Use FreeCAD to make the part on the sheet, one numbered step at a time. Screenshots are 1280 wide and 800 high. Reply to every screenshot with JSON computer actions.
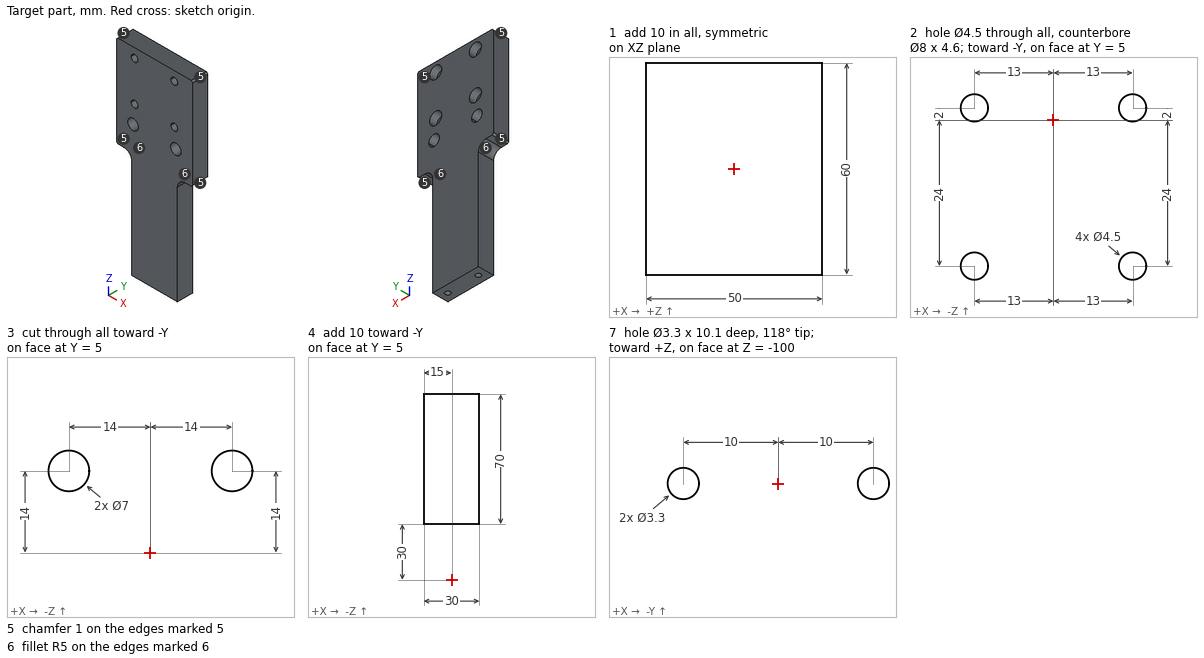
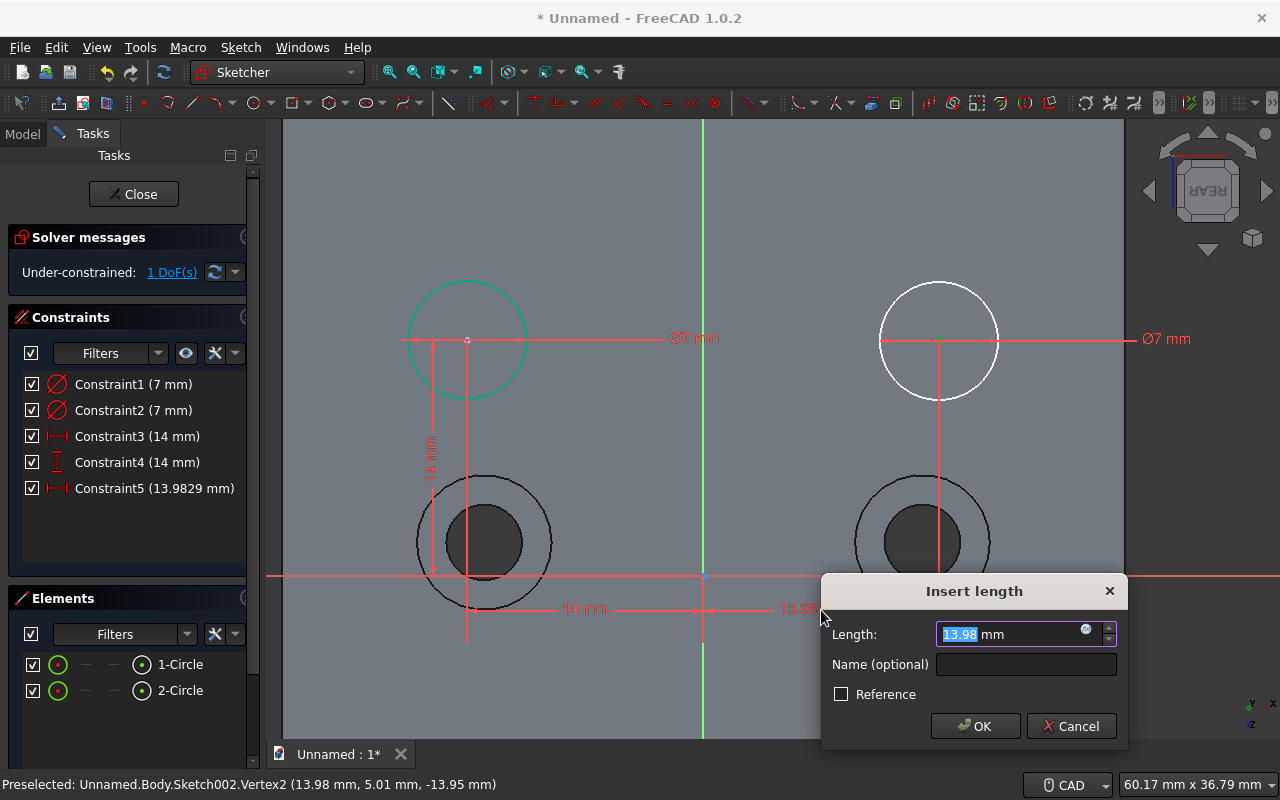
{"action": "type", "text": "14"}
{"action": "key", "text": "Return"}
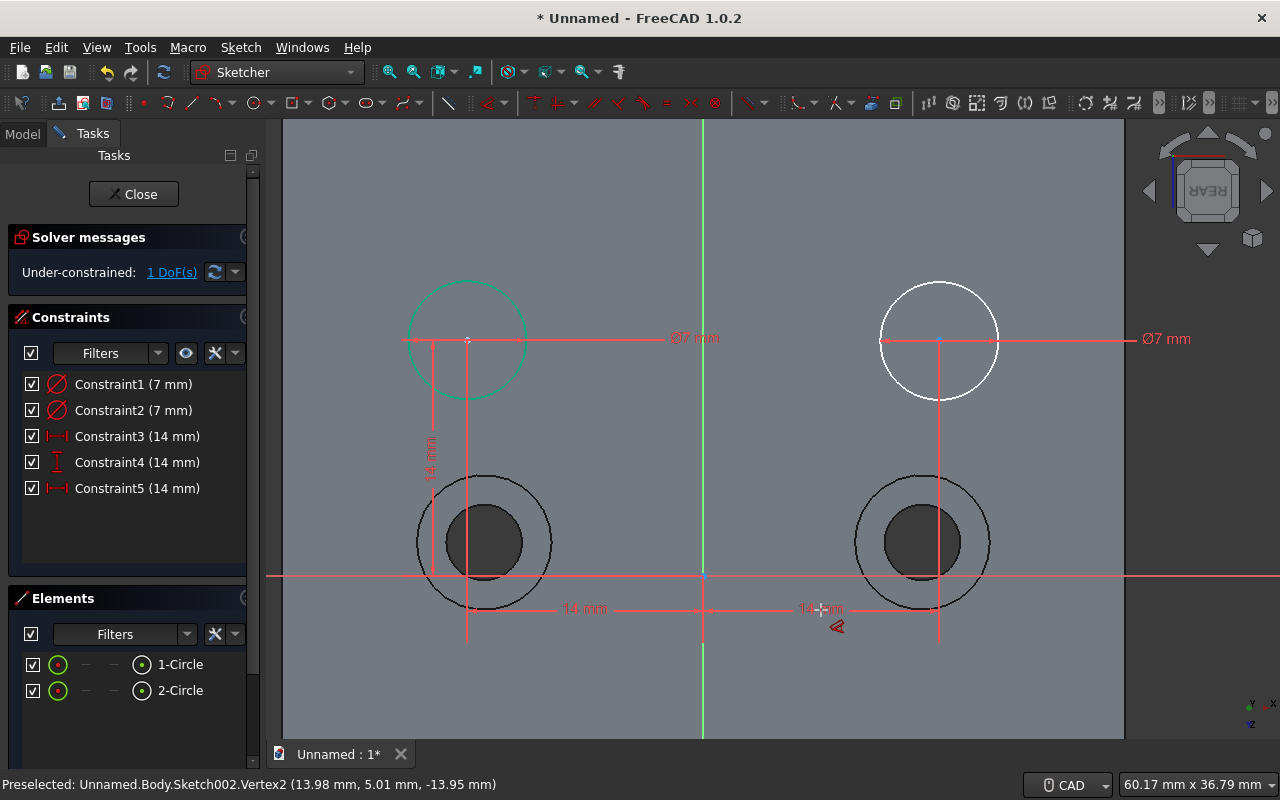
{"action": "left_click", "coordinate": [939, 341]}
{"action": "left_click", "coordinate": [973, 459]}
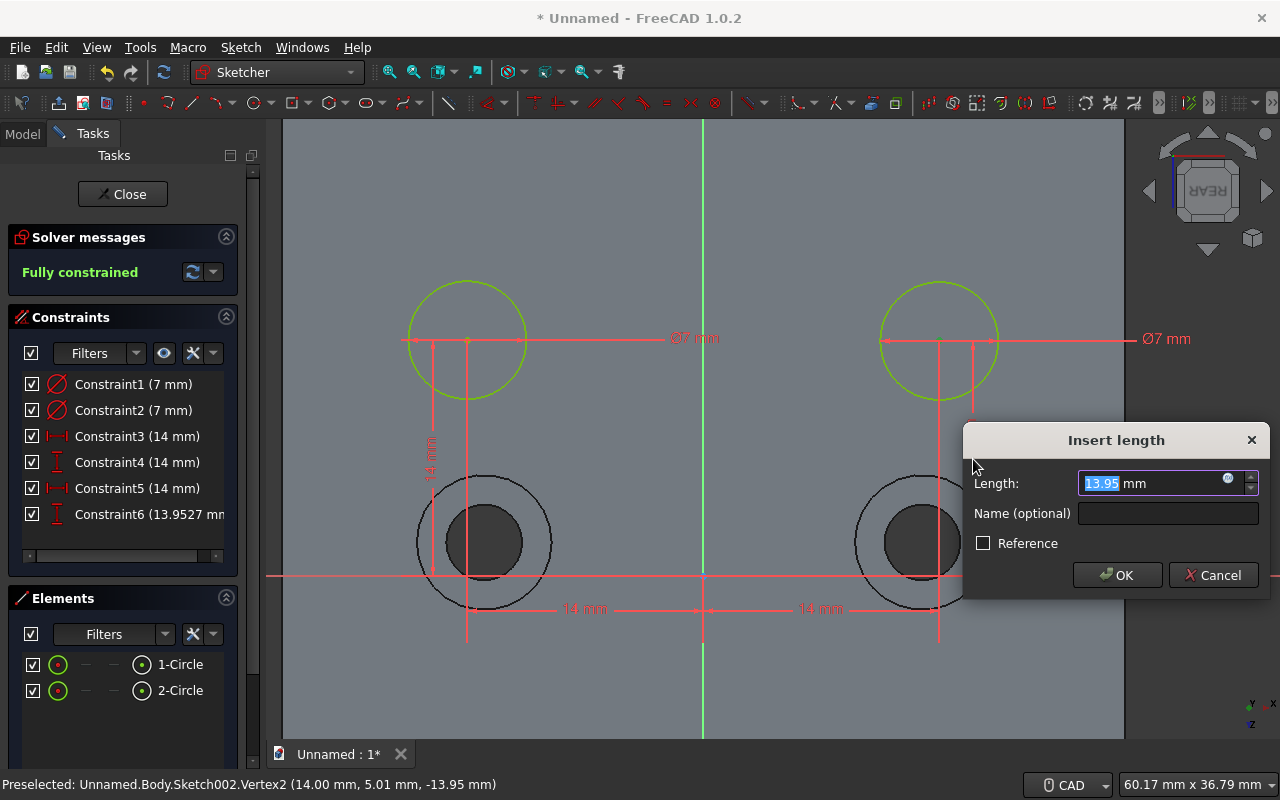
{"action": "type", "text": "14"}
{"action": "key", "text": "Return"}
{"action": "key", "text": "Escape"}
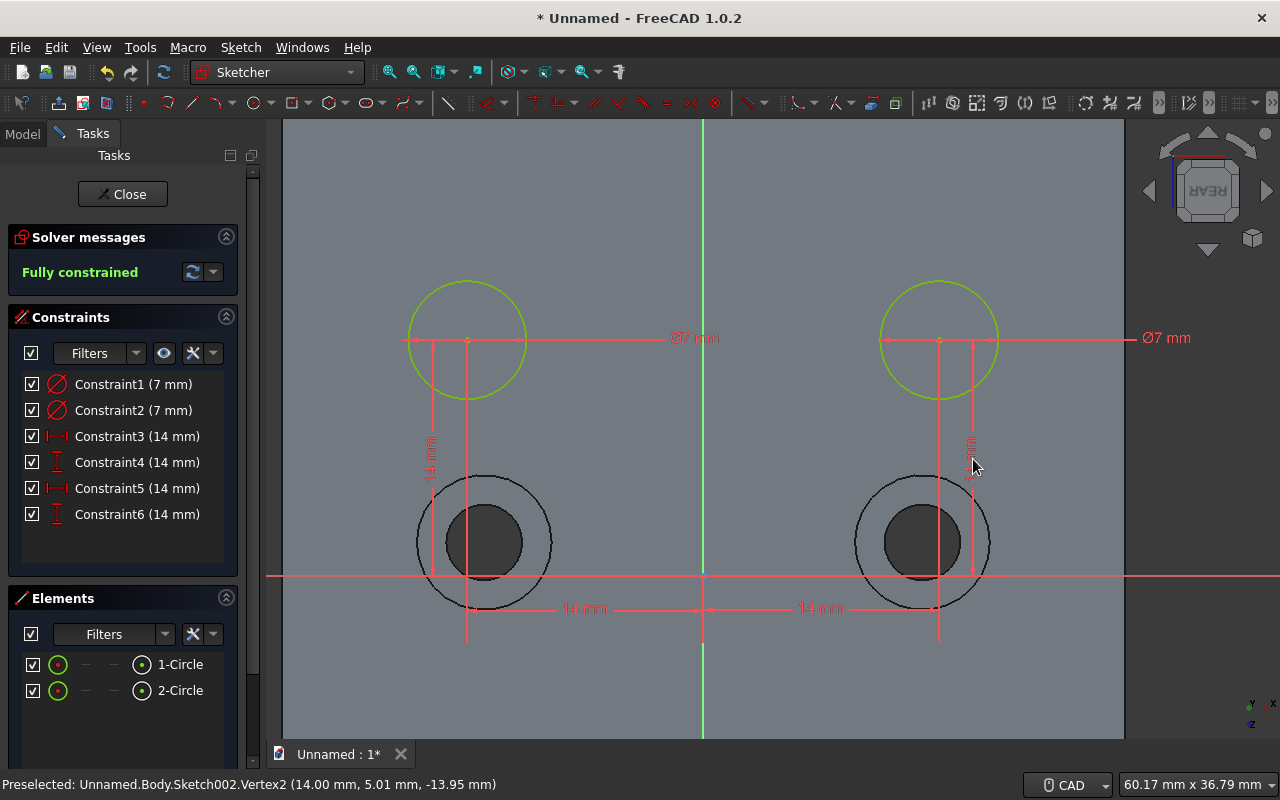
{"action": "left_click", "coordinate": [123, 194]}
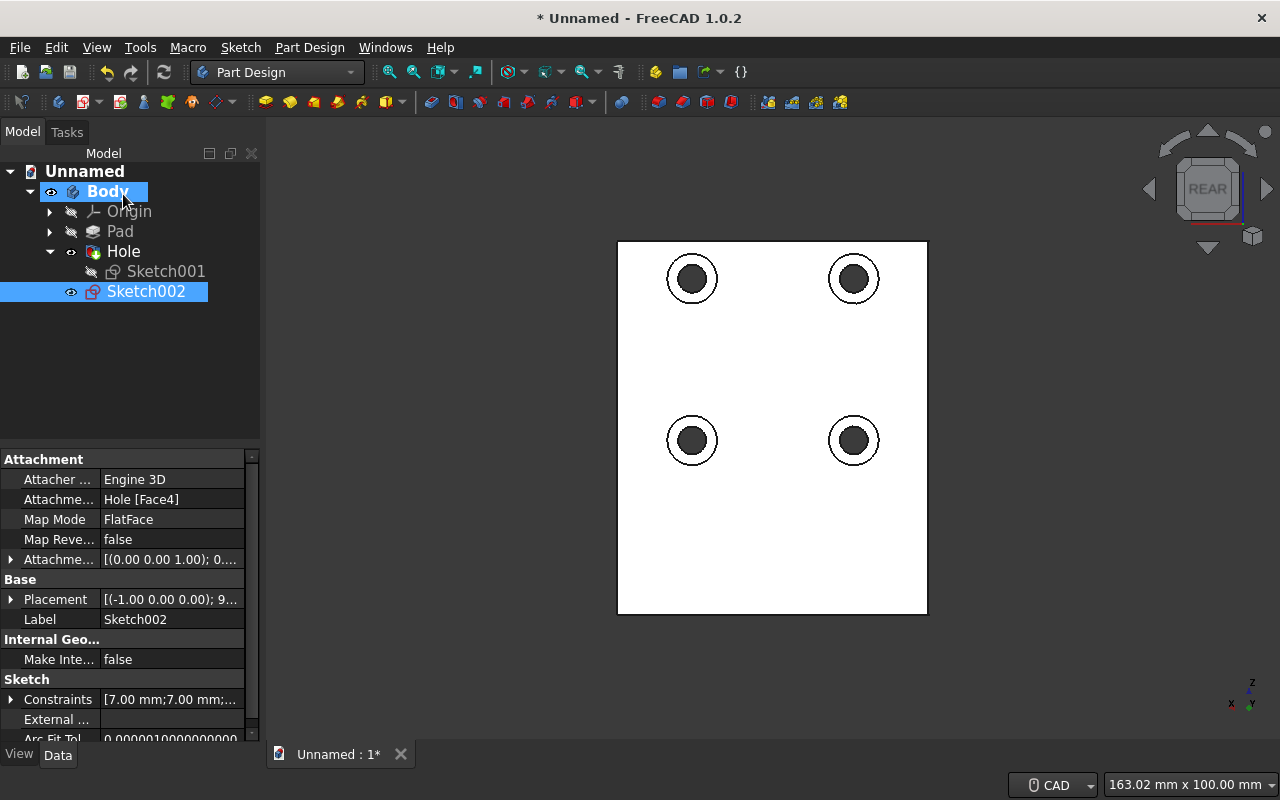
{"action": "left_click", "coordinate": [432, 102]}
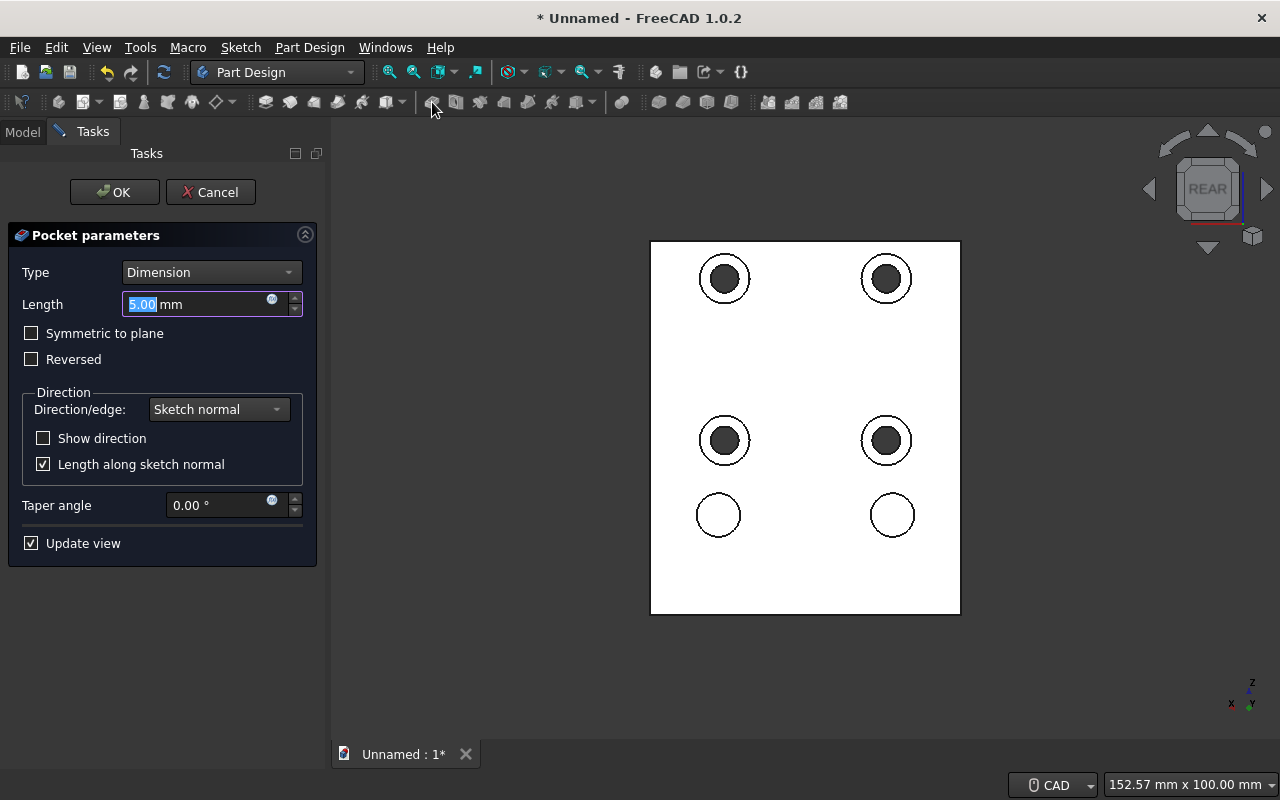
{"action": "left_click", "coordinate": [212, 272]}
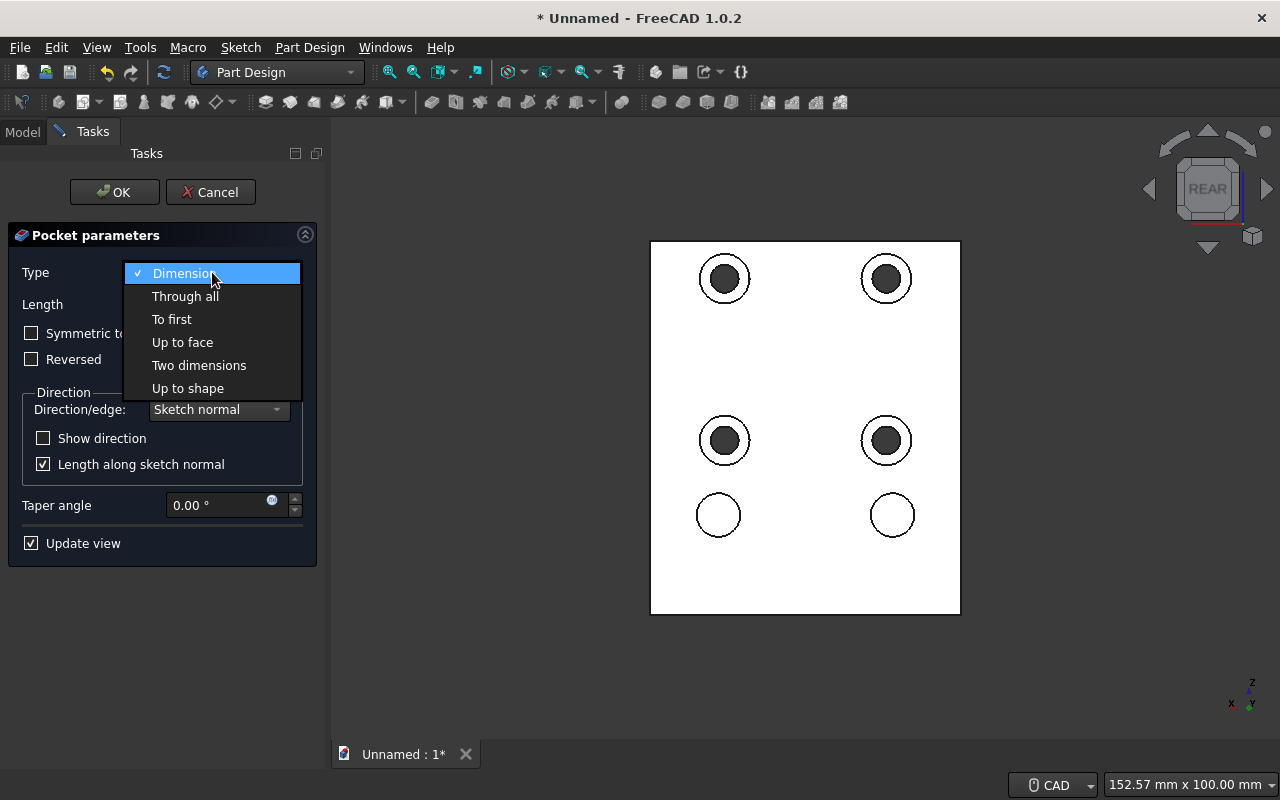
{"action": "left_click", "coordinate": [212, 296]}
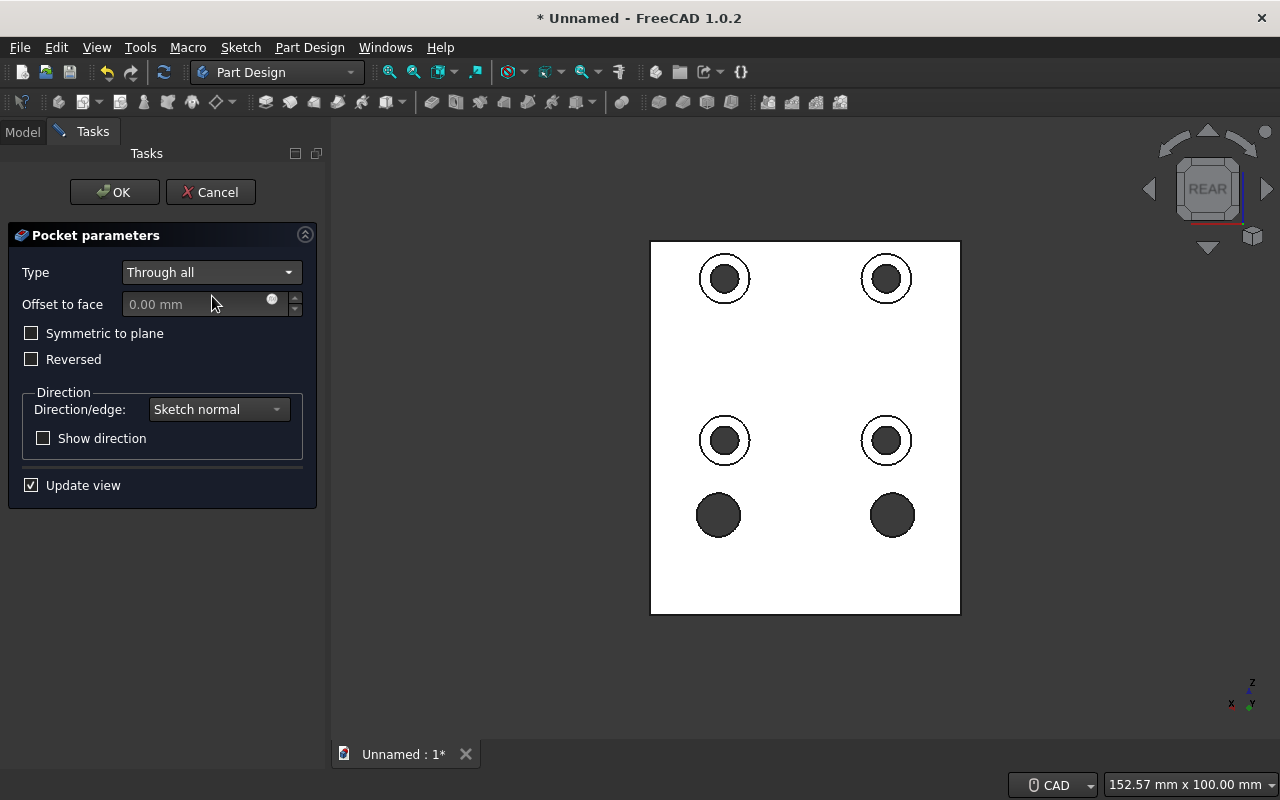
{"action": "left_click", "coordinate": [115, 192]}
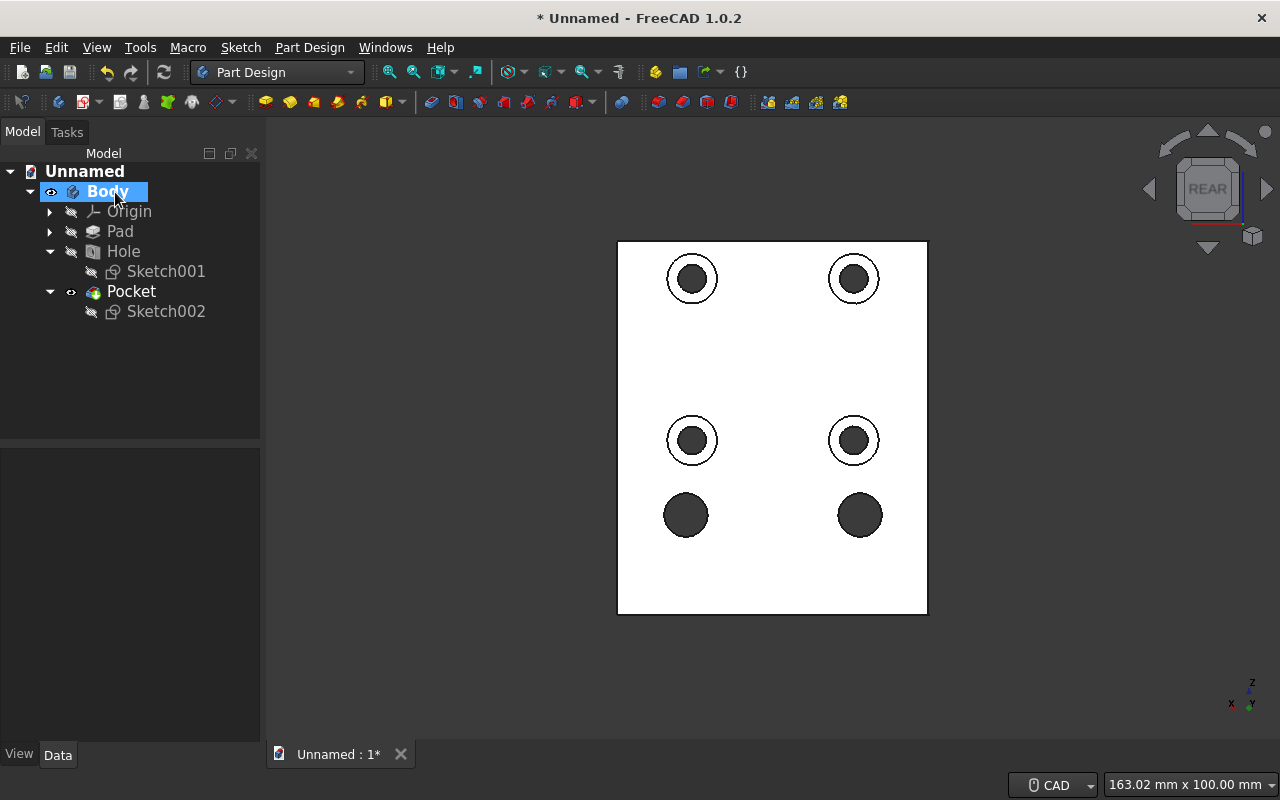
{"action": "left_click", "coordinate": [773, 374]}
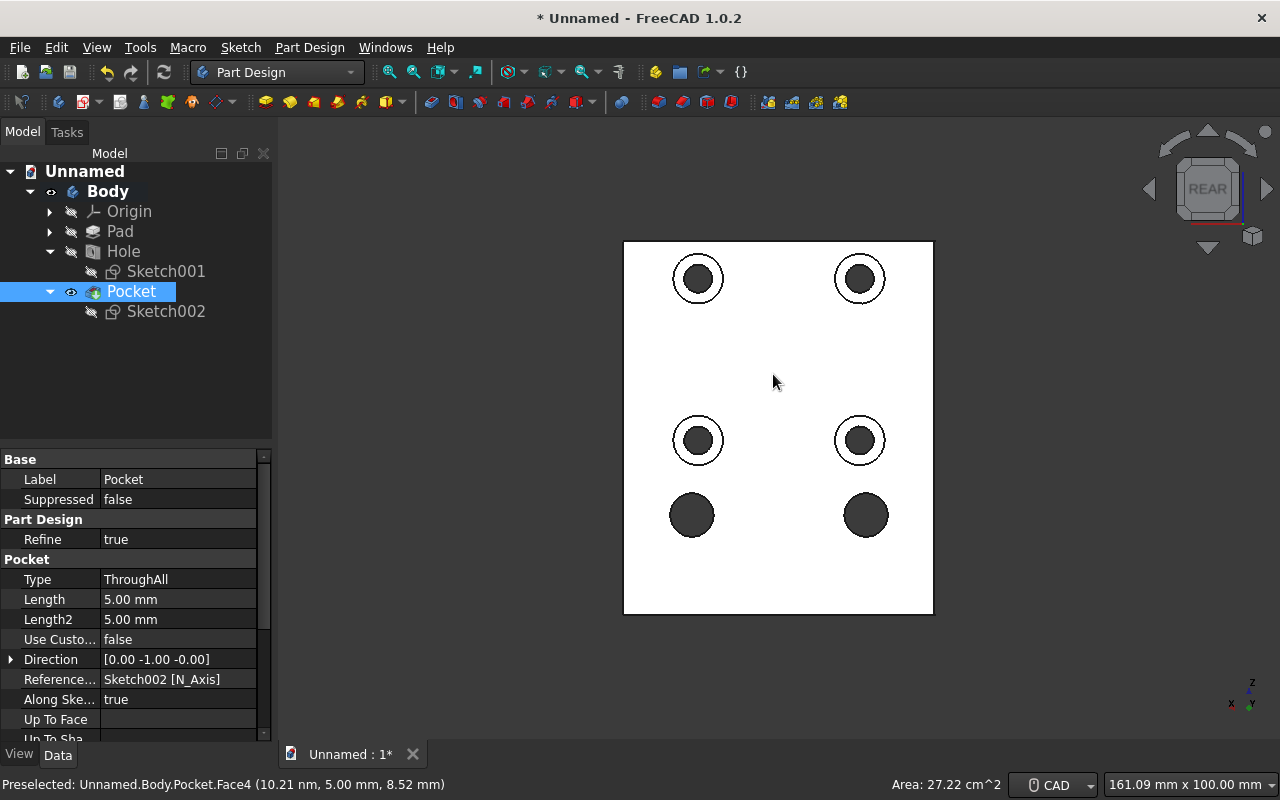
{"action": "left_click", "coordinate": [84, 102]}